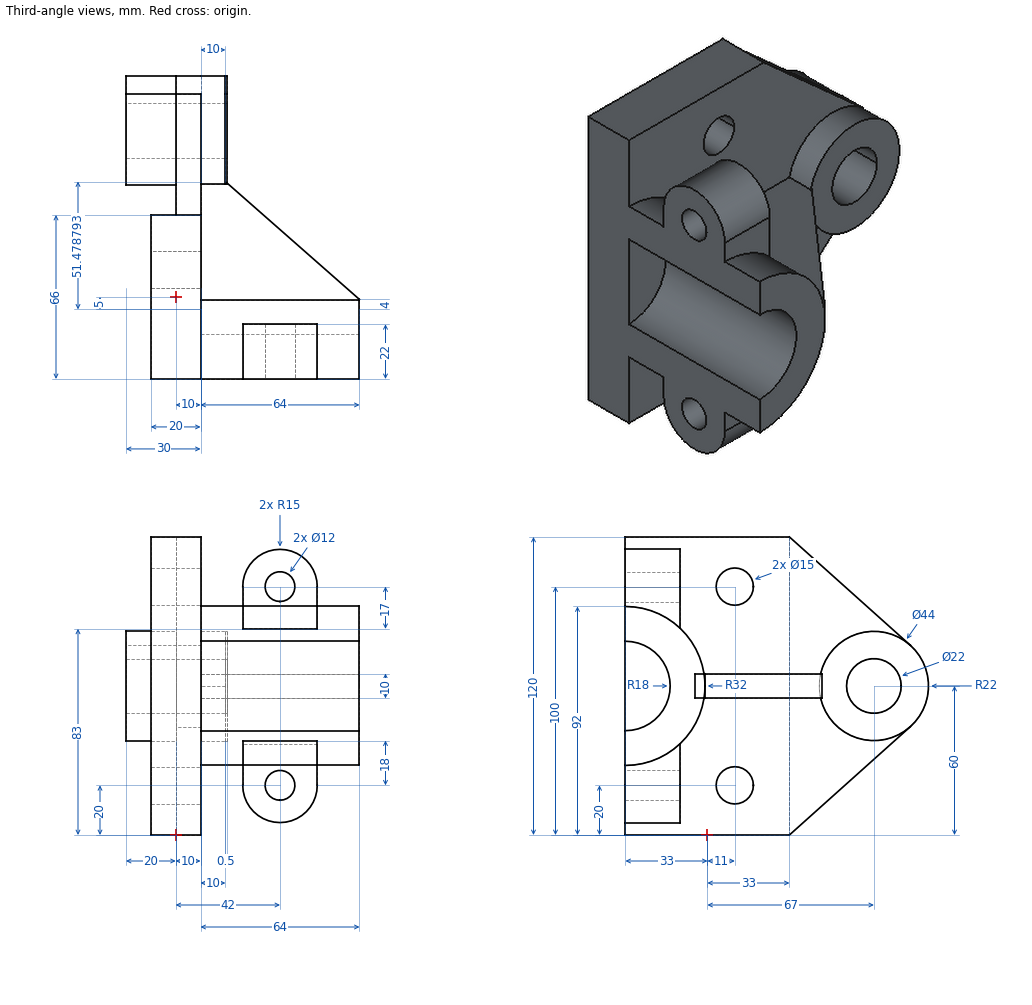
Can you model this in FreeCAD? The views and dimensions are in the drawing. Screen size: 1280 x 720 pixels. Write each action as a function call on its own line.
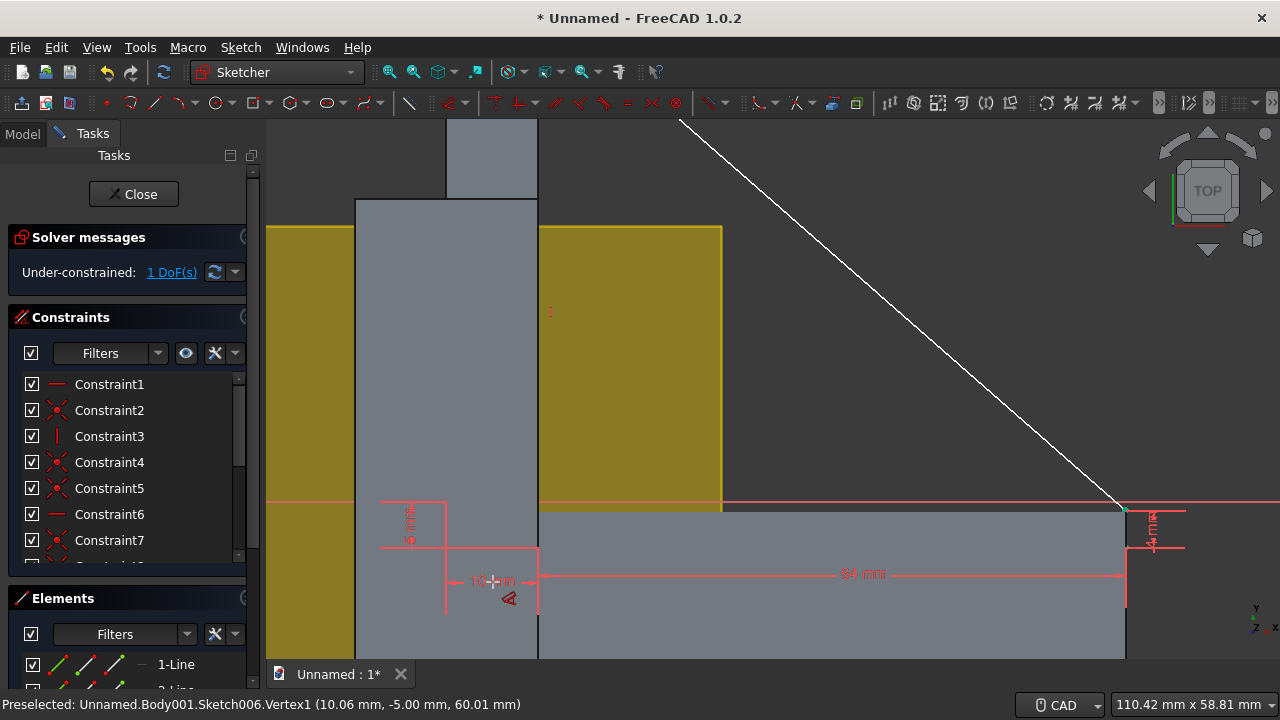
click(538, 218)
click(504, 347)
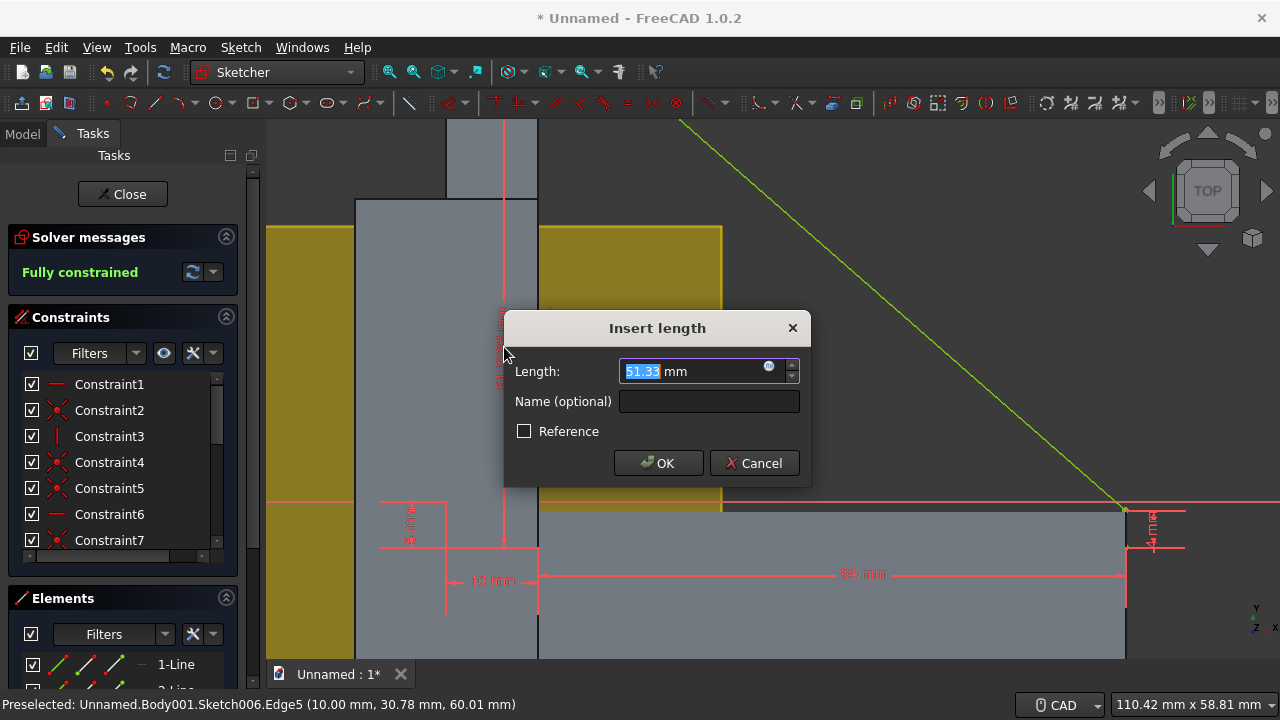
text(51.478793)
key(Return)
key(Escape)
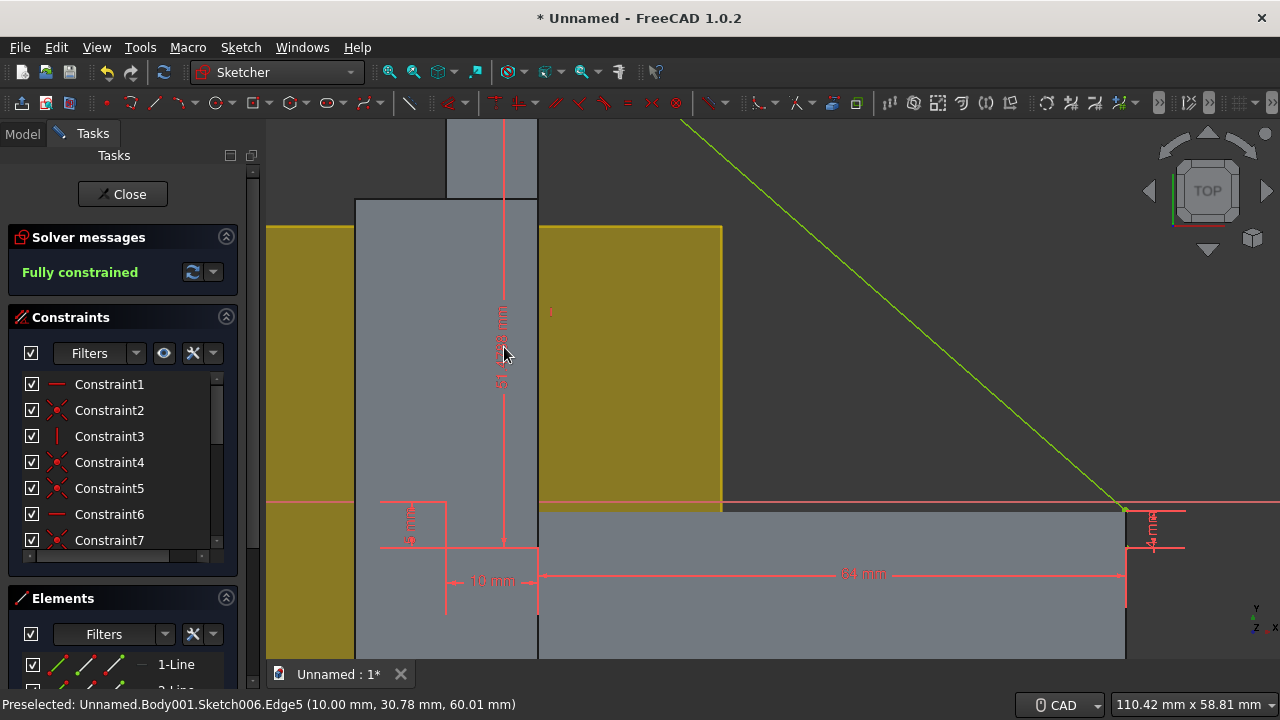
click(123, 194)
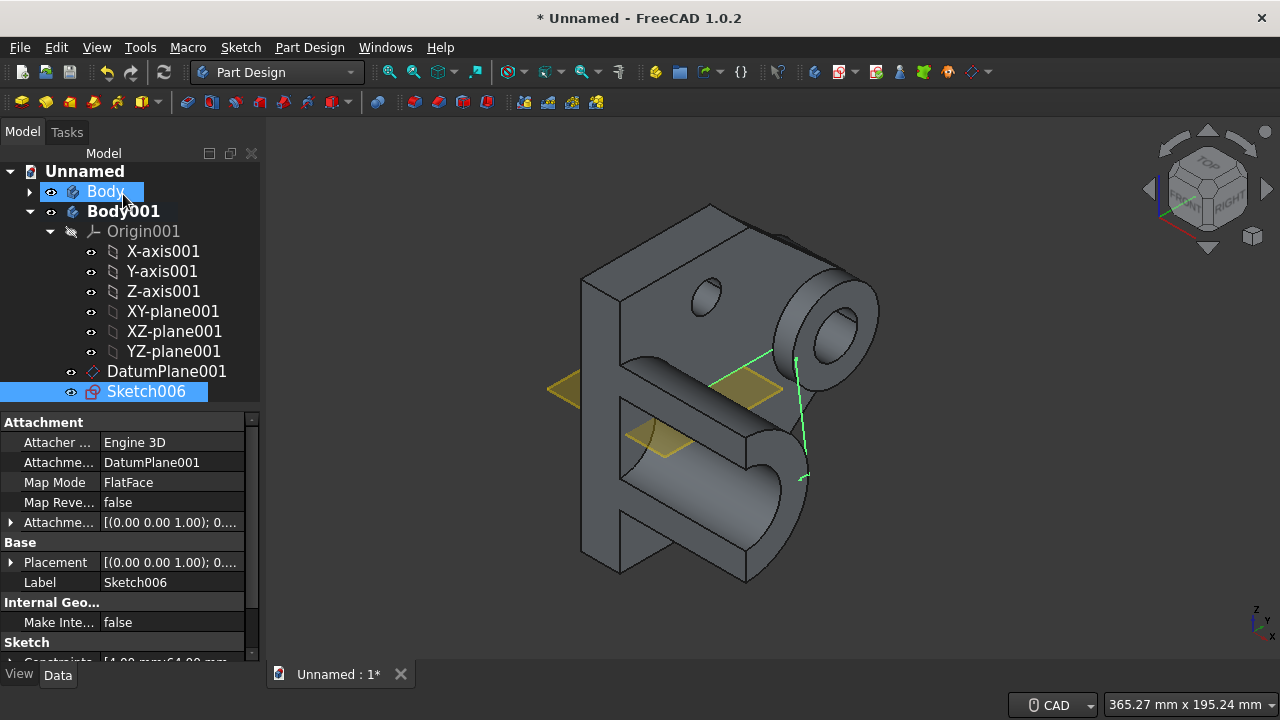
click(22, 102)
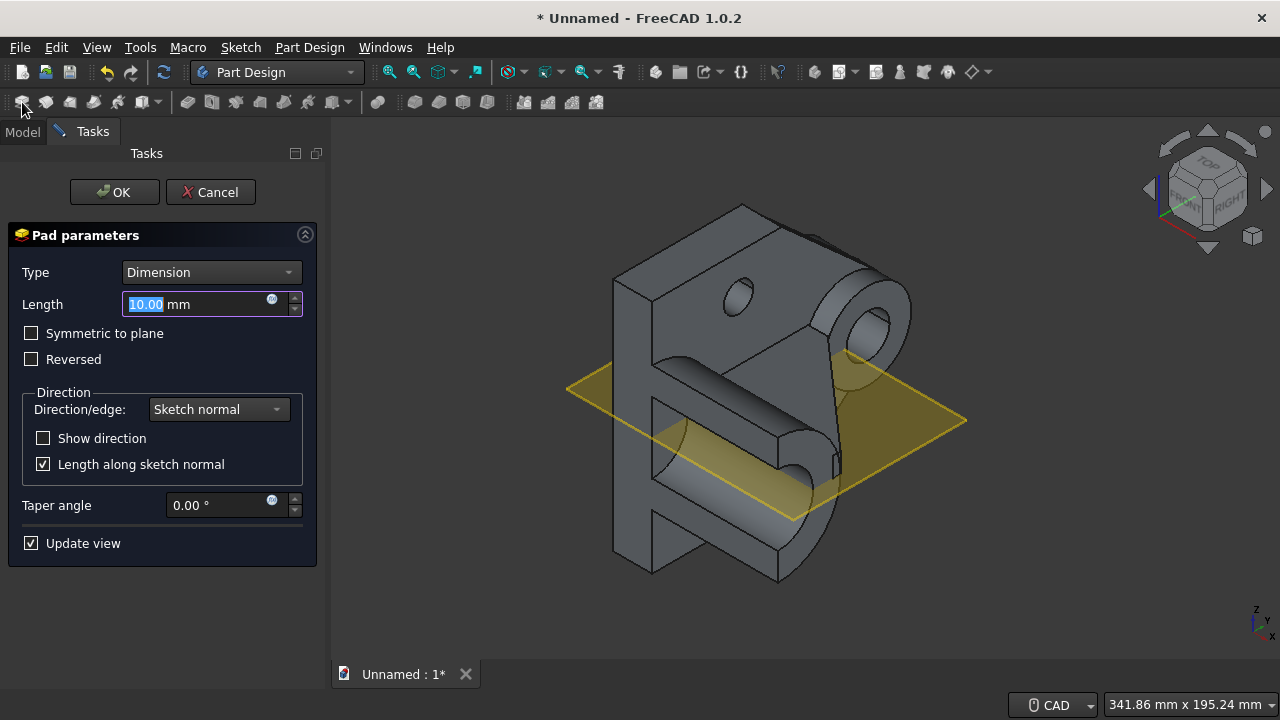
text(10)
key(Tab)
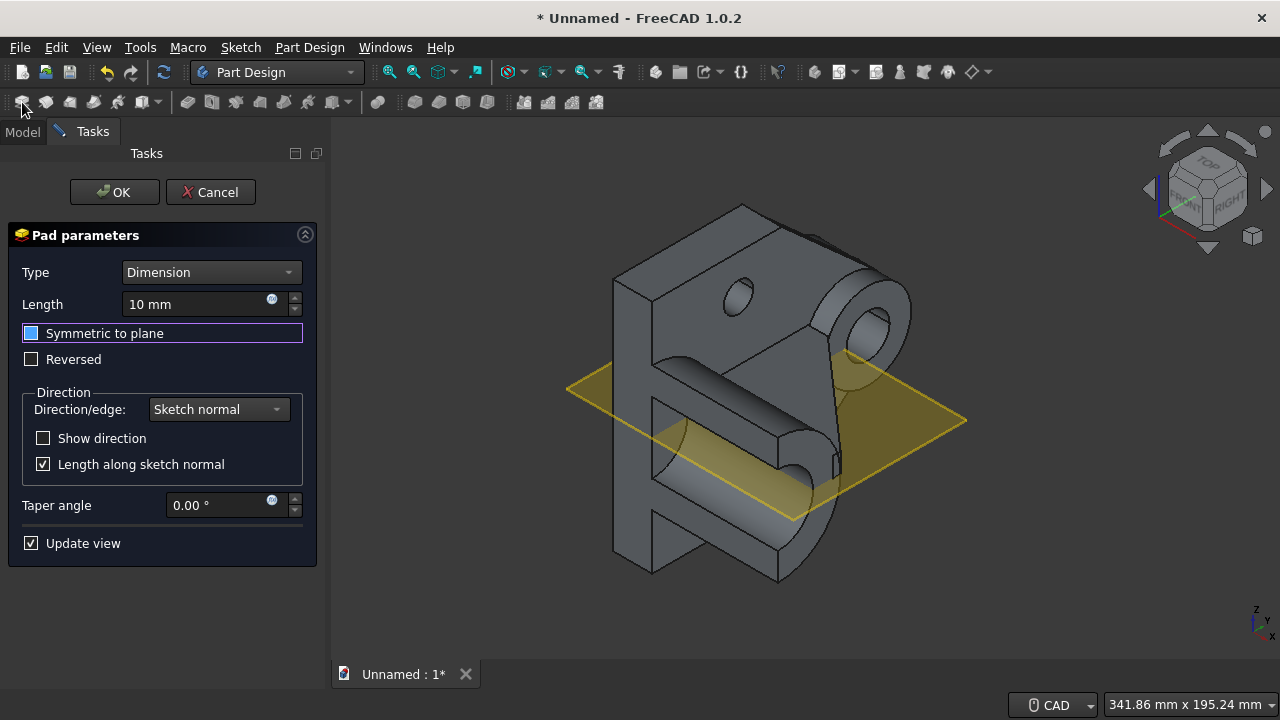
click(30, 333)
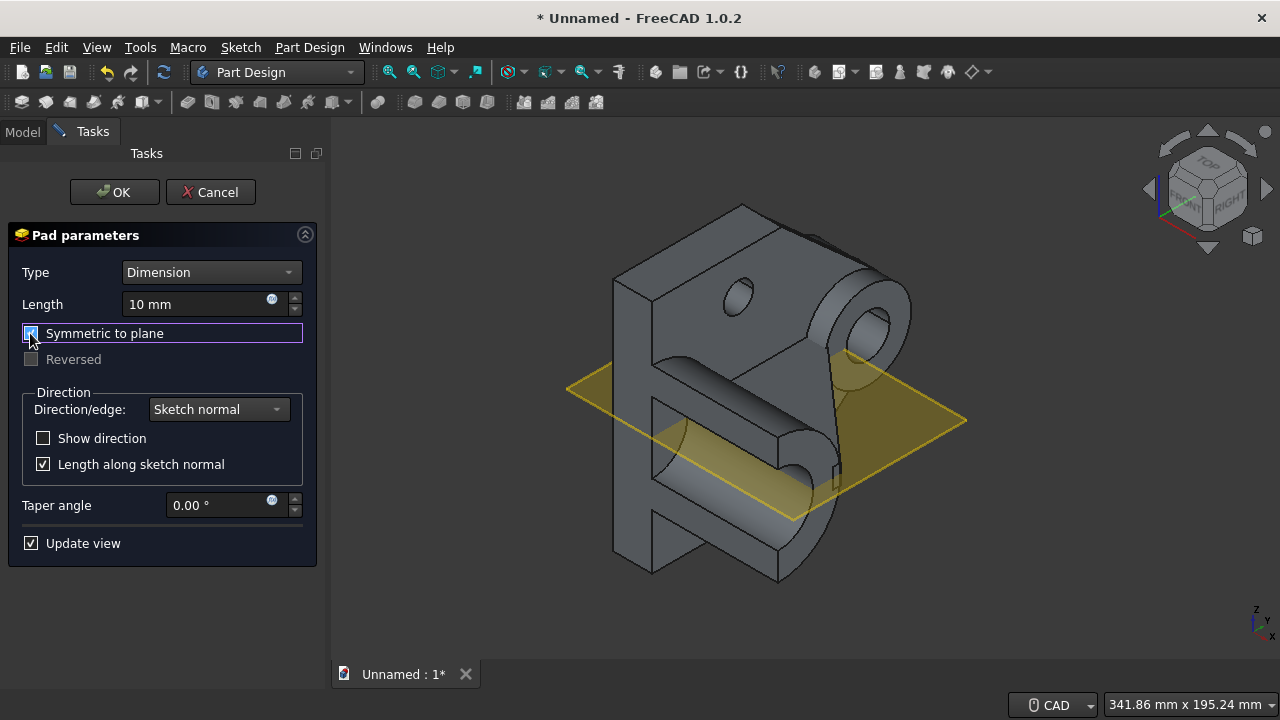
click(115, 192)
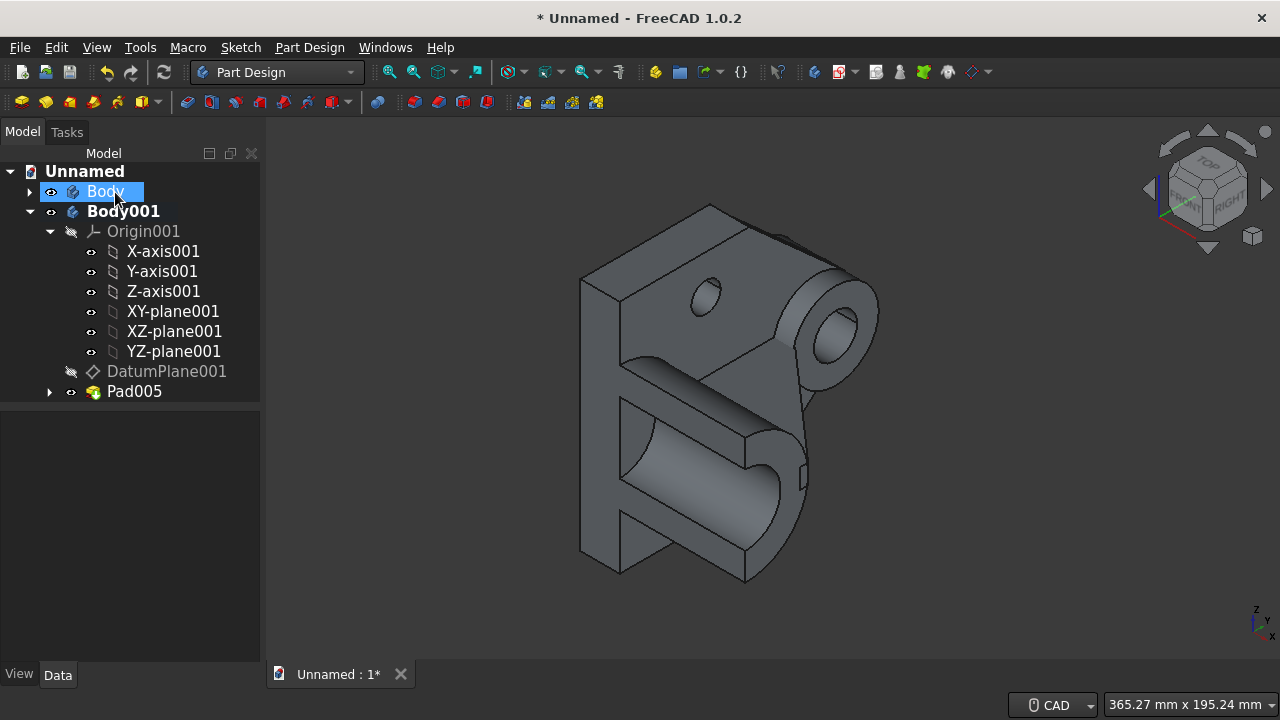
click(390, 72)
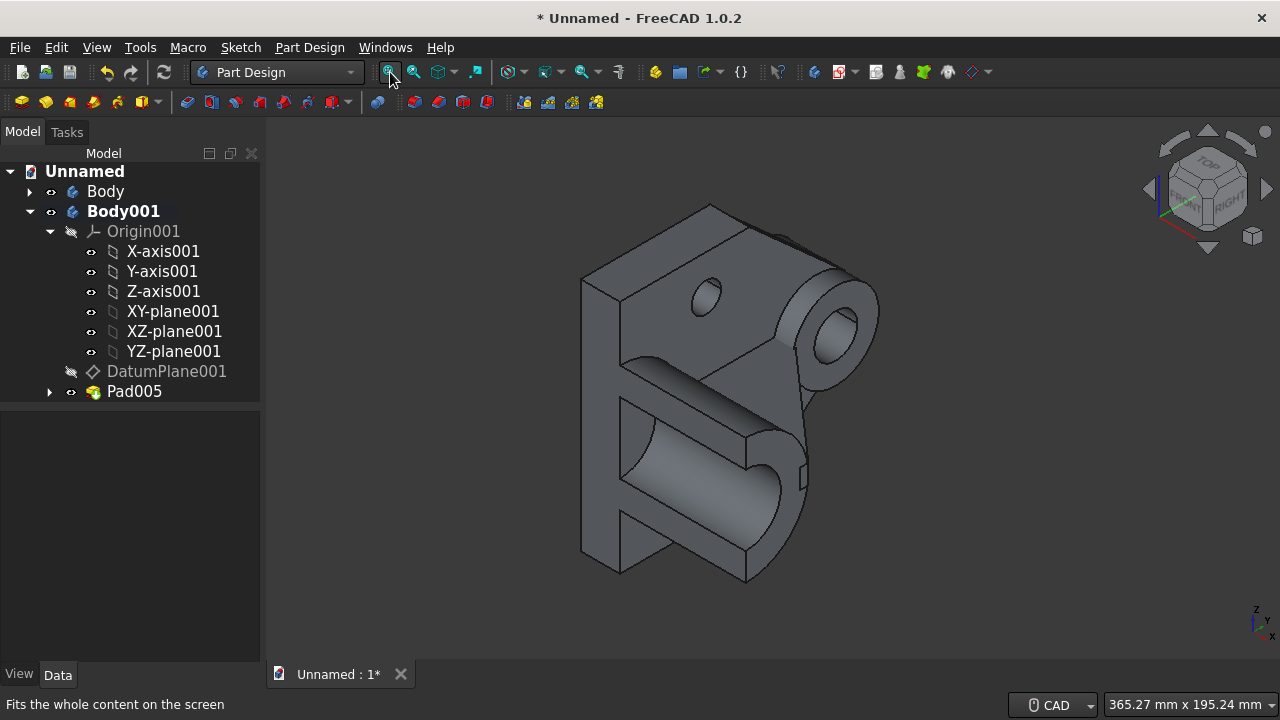
double_click(96, 192)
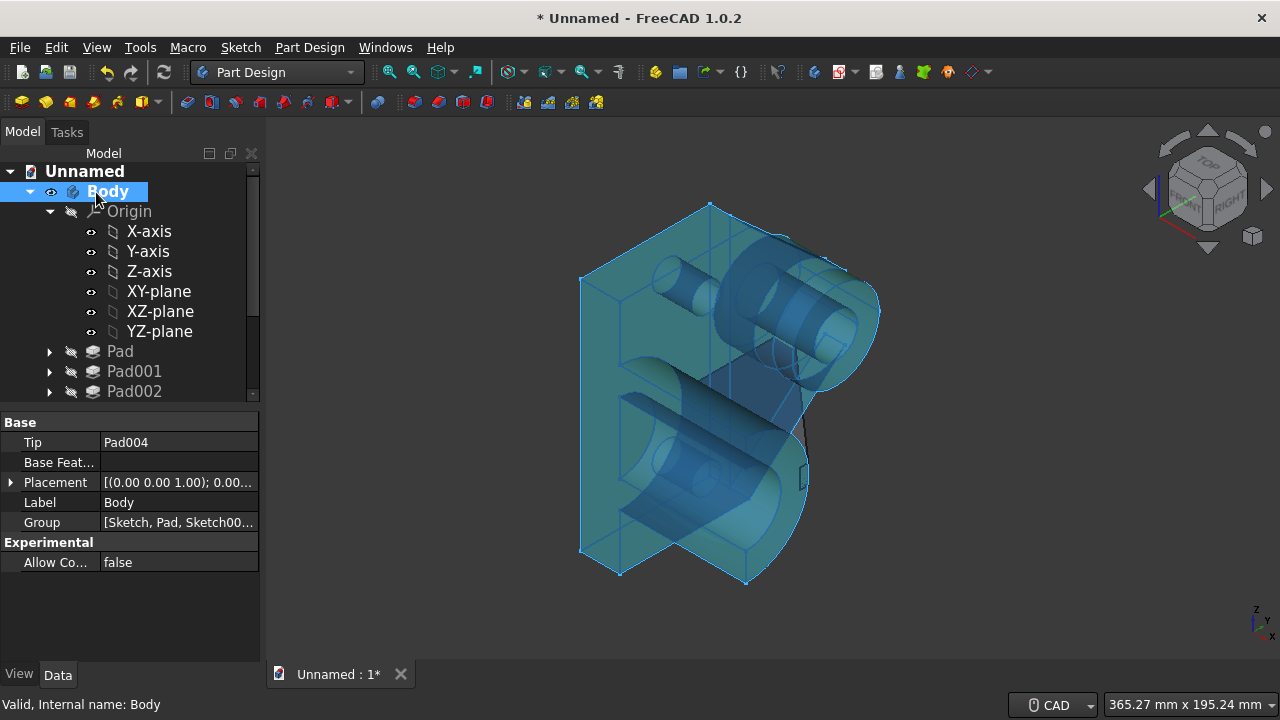
scroll(100, 287, down, 3)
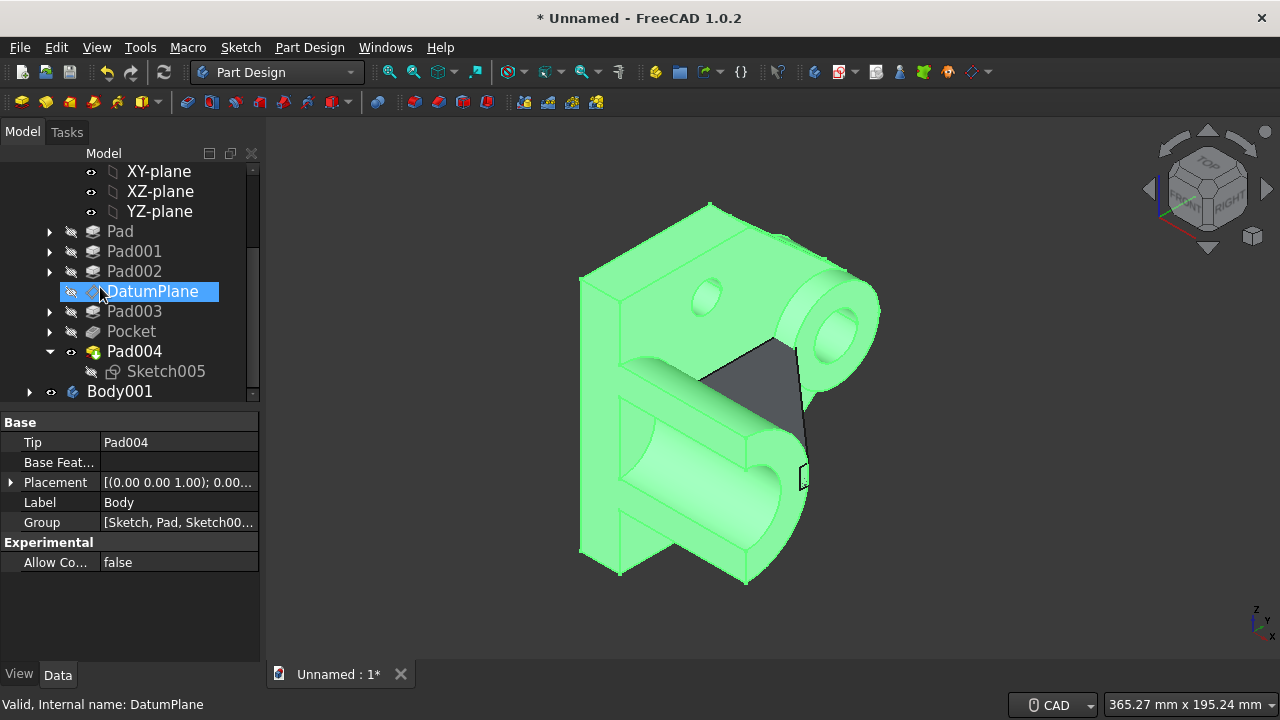
click(96, 392)